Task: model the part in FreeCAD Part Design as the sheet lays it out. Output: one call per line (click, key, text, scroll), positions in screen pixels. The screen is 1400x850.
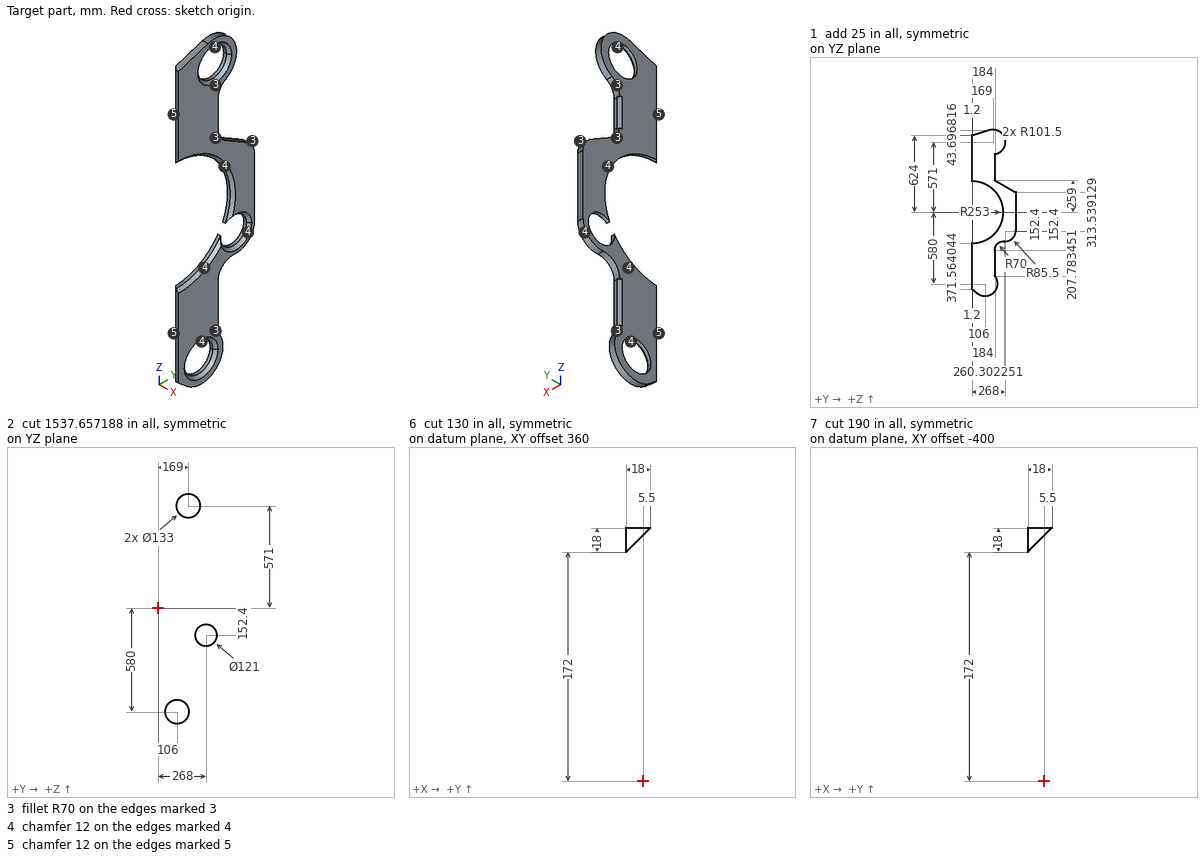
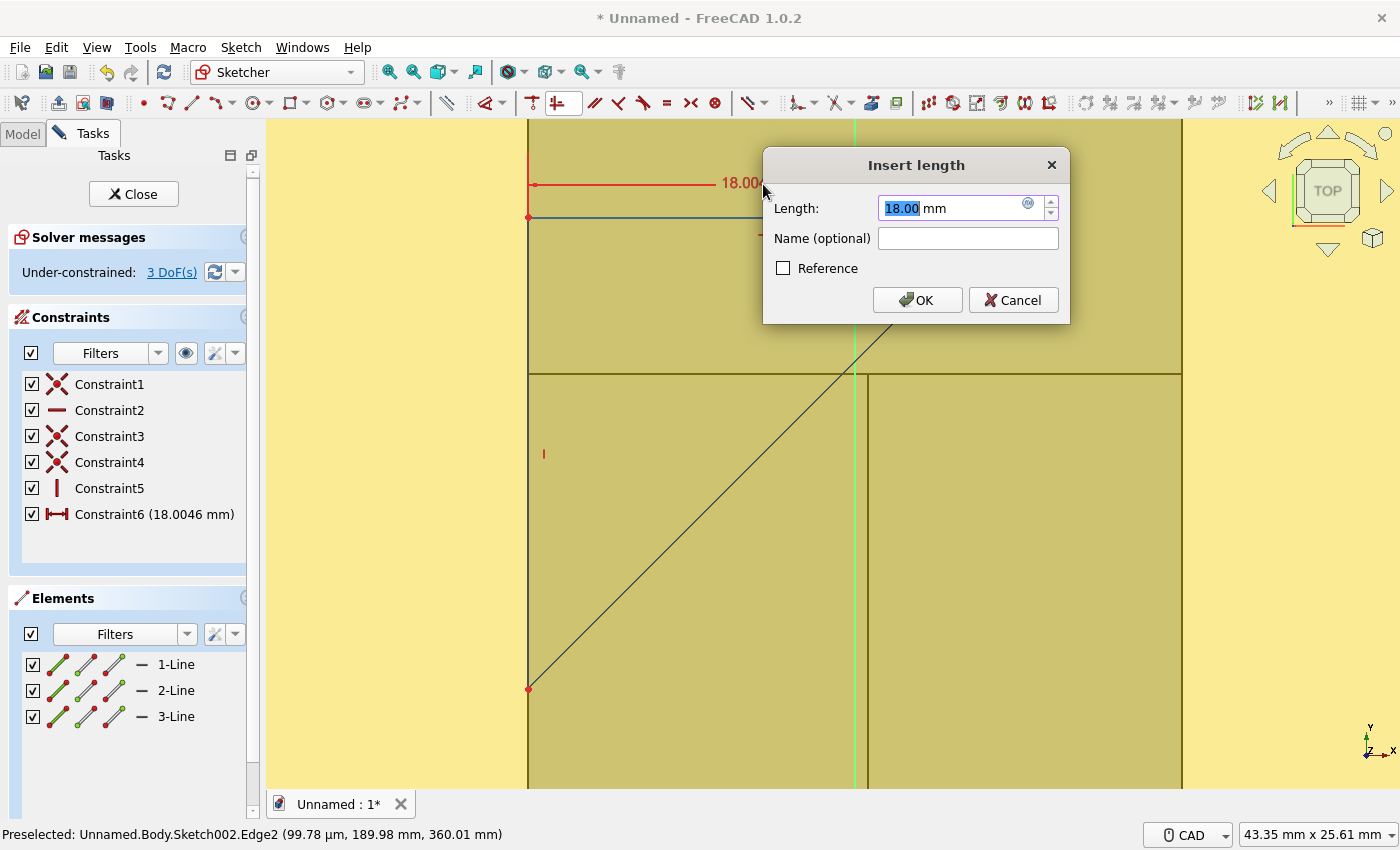
text(18)
key(Return)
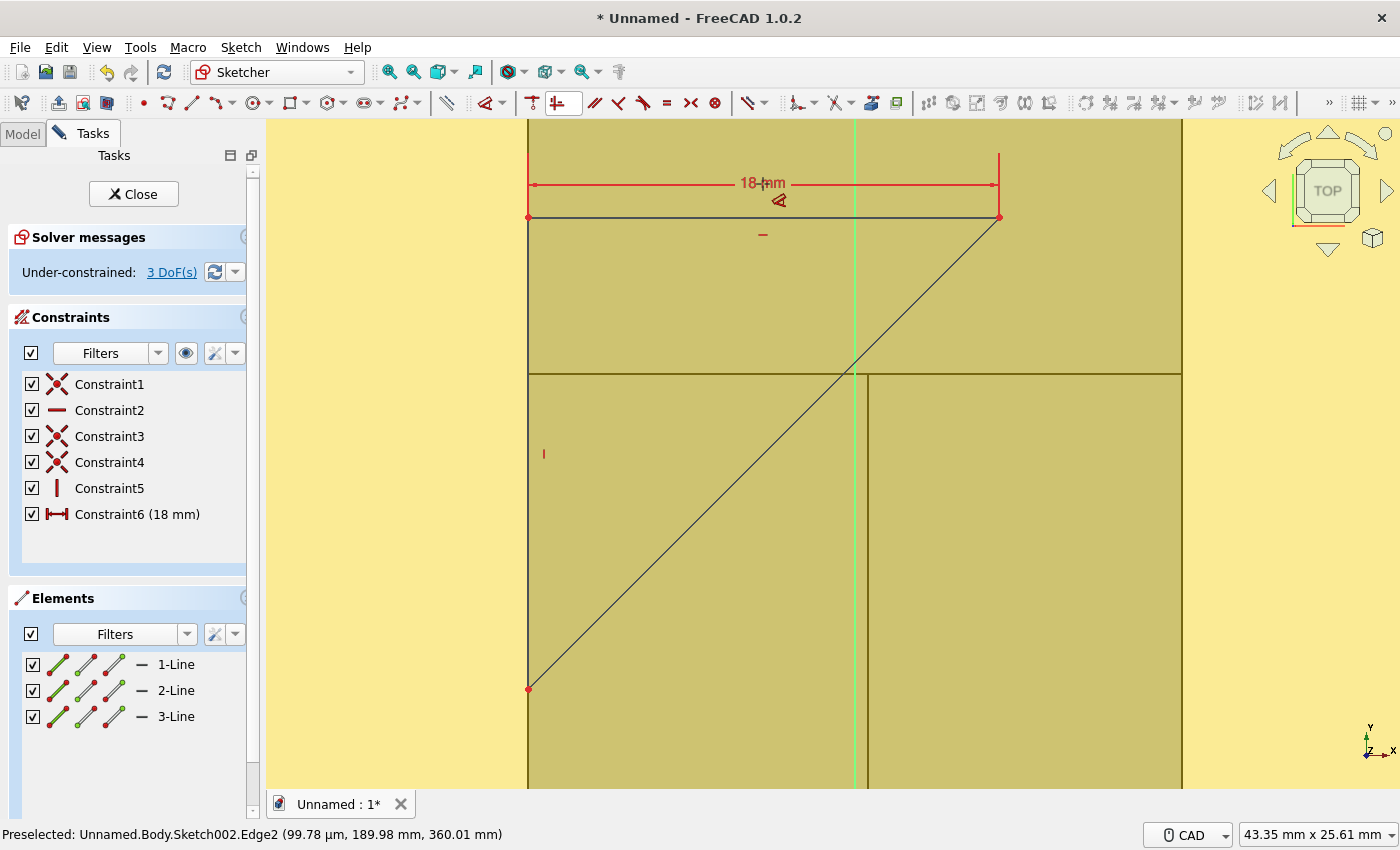
click(528, 359)
click(494, 454)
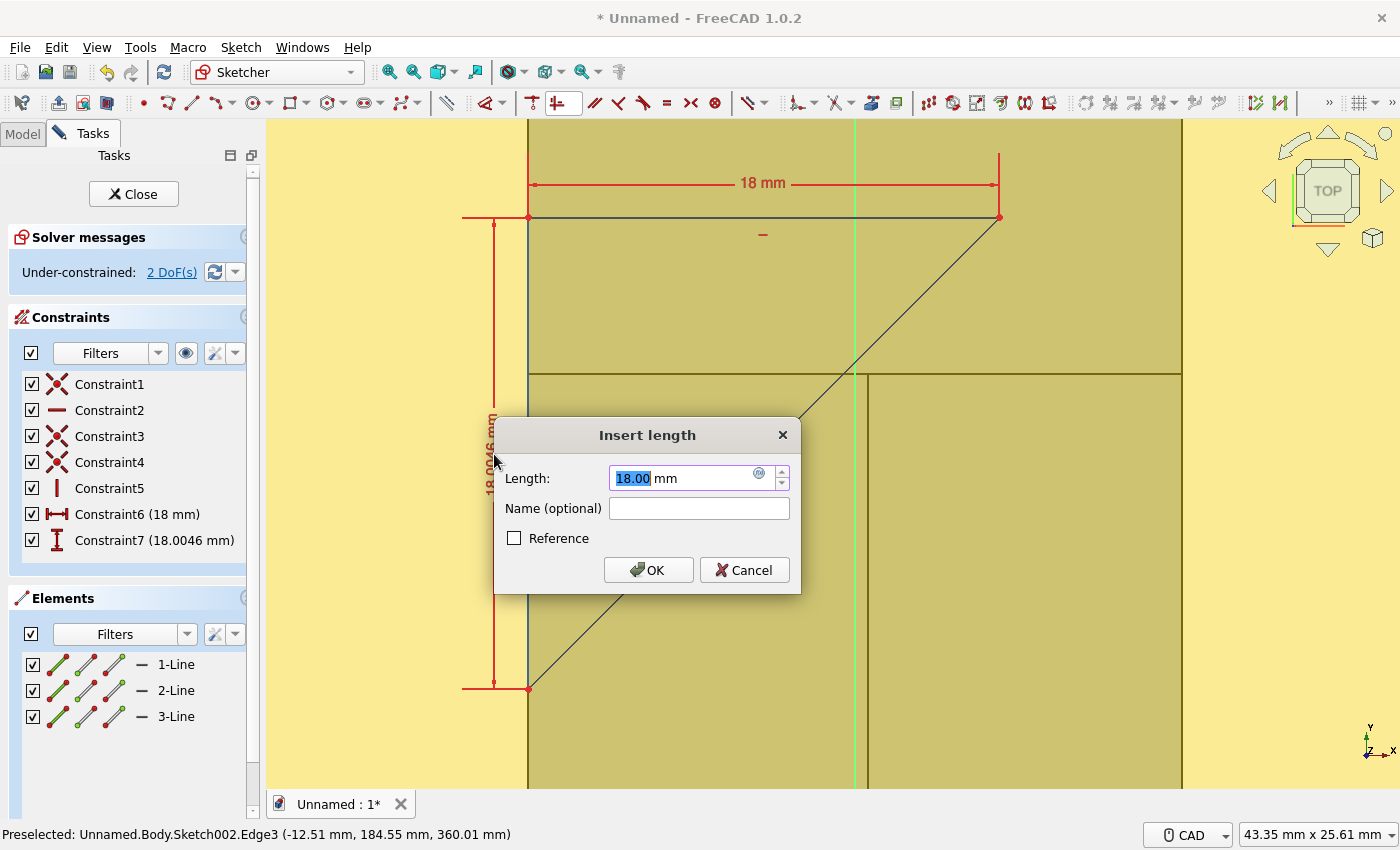
text(18)
key(Return)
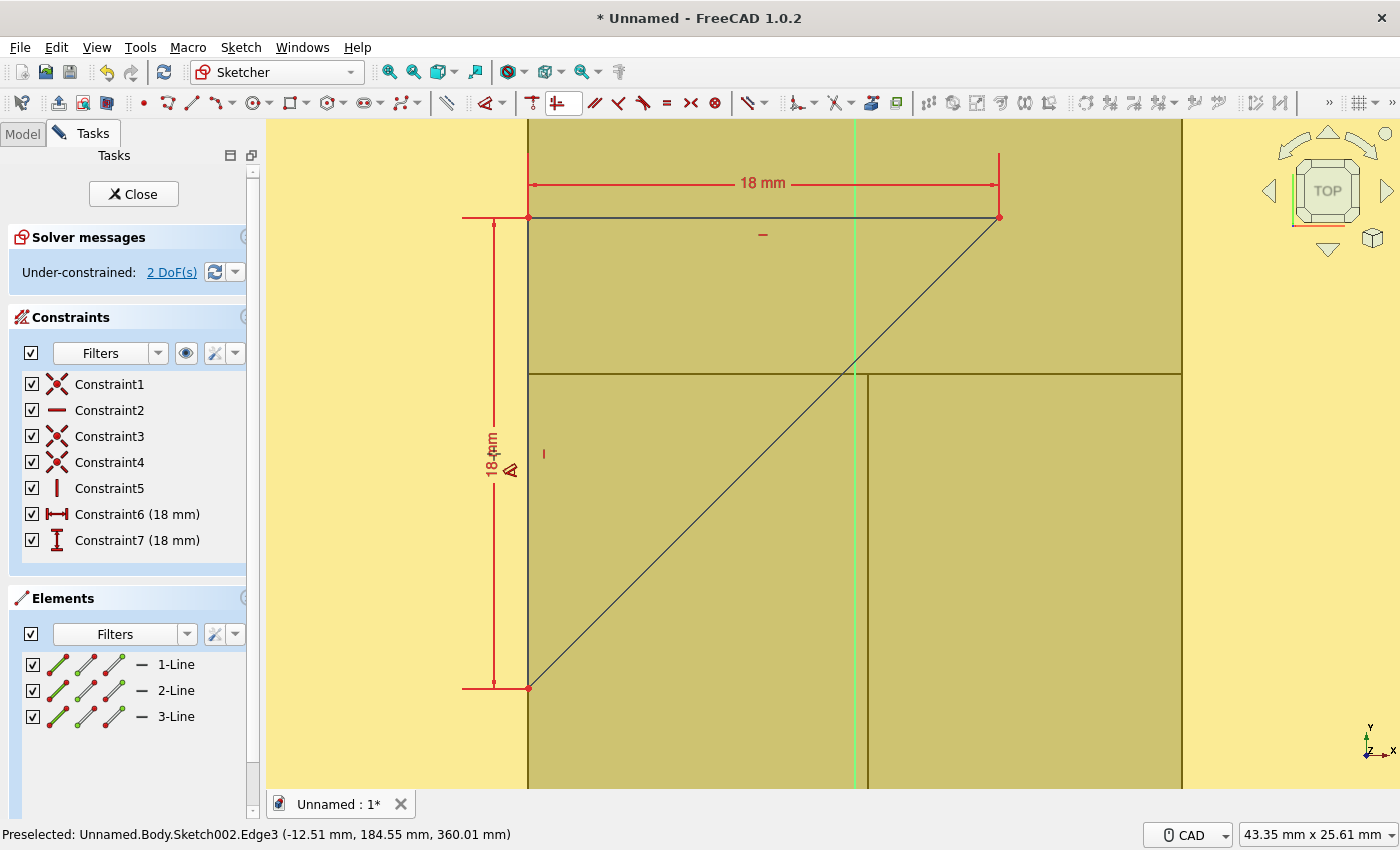
click(528, 689)
click(494, 725)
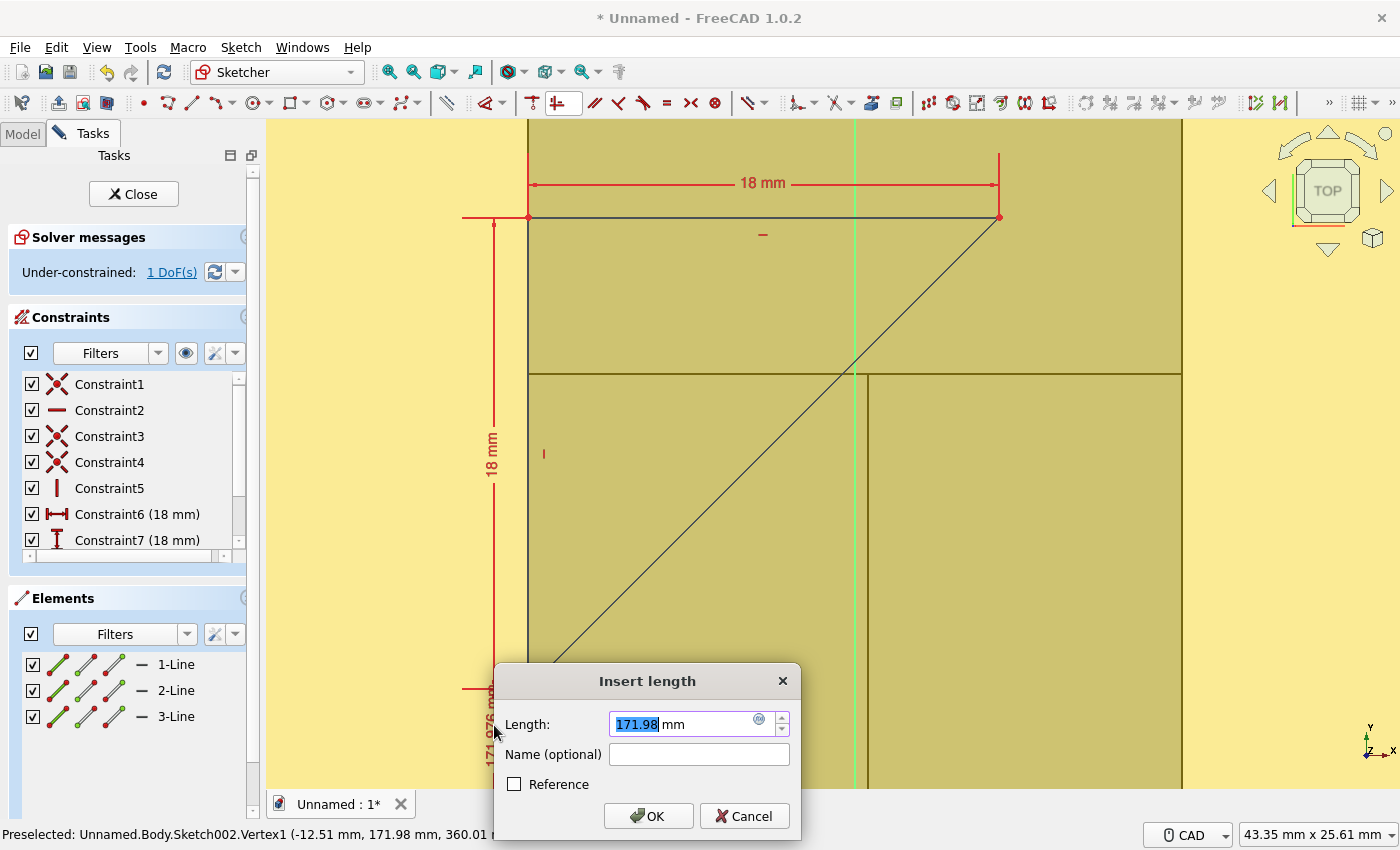
text(172)
key(Return)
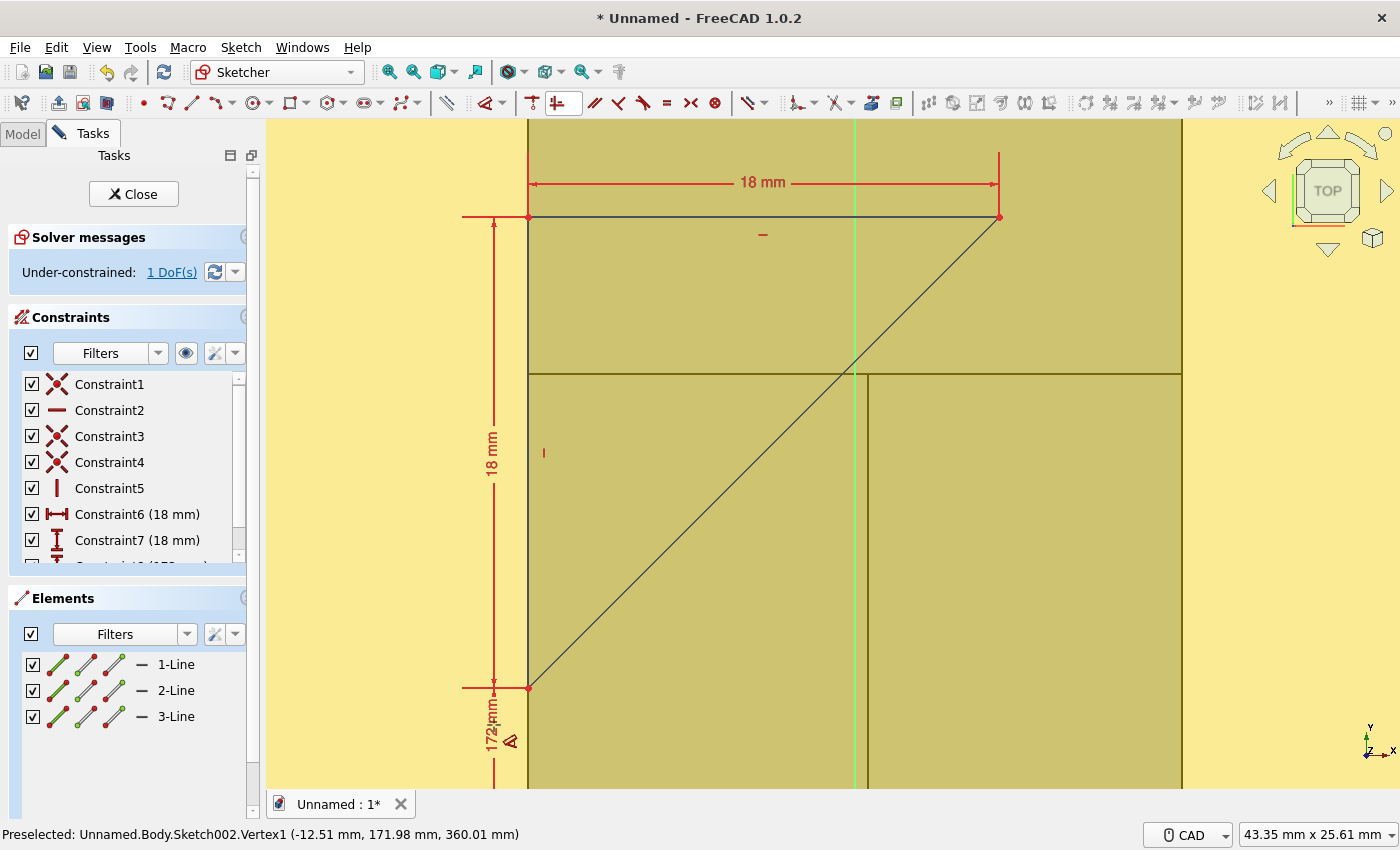
click(999, 217)
click(927, 183)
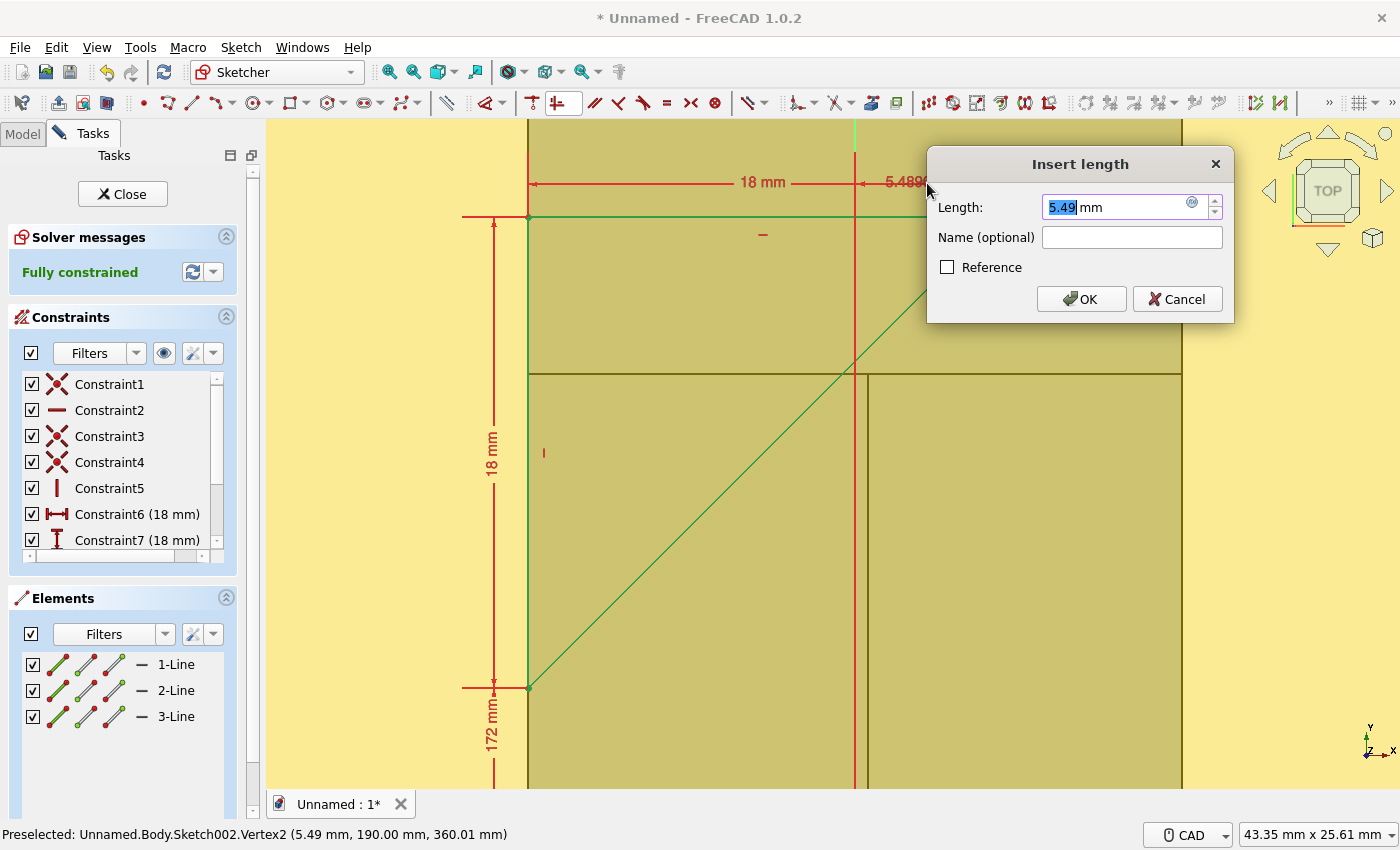
text(5.5)
key(Return)
key(Escape)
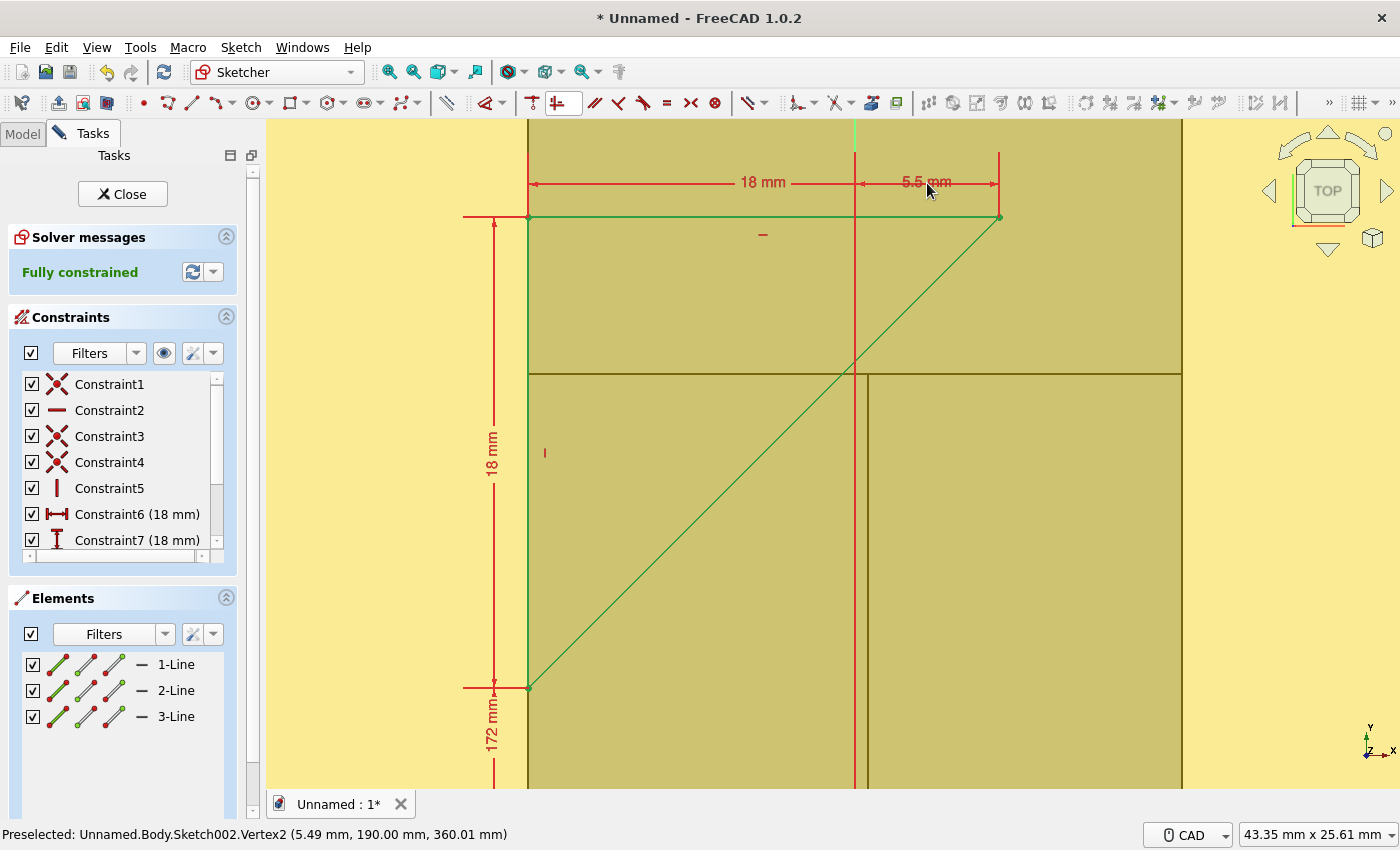
click(123, 194)